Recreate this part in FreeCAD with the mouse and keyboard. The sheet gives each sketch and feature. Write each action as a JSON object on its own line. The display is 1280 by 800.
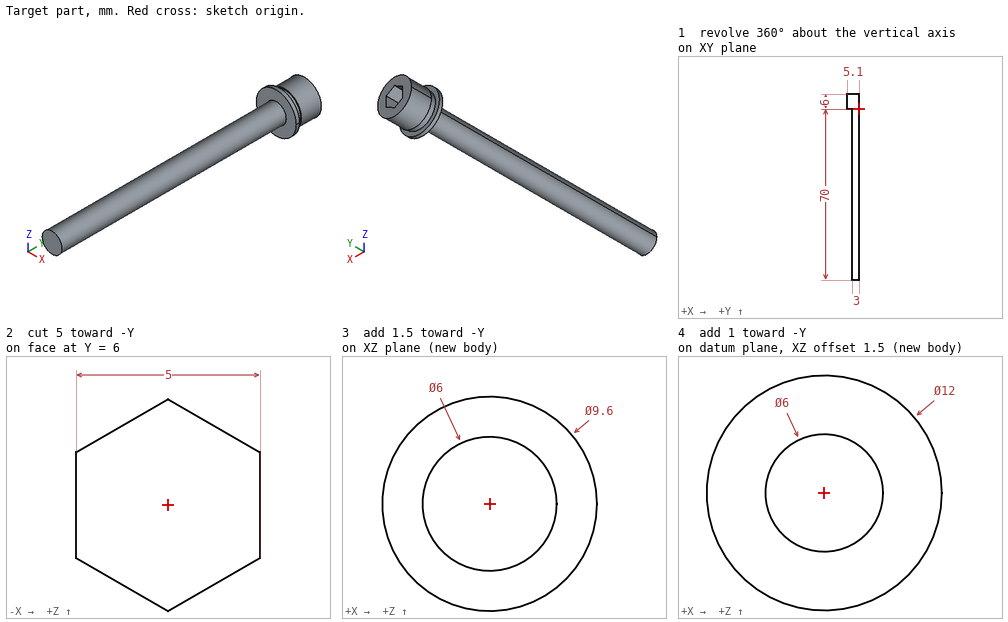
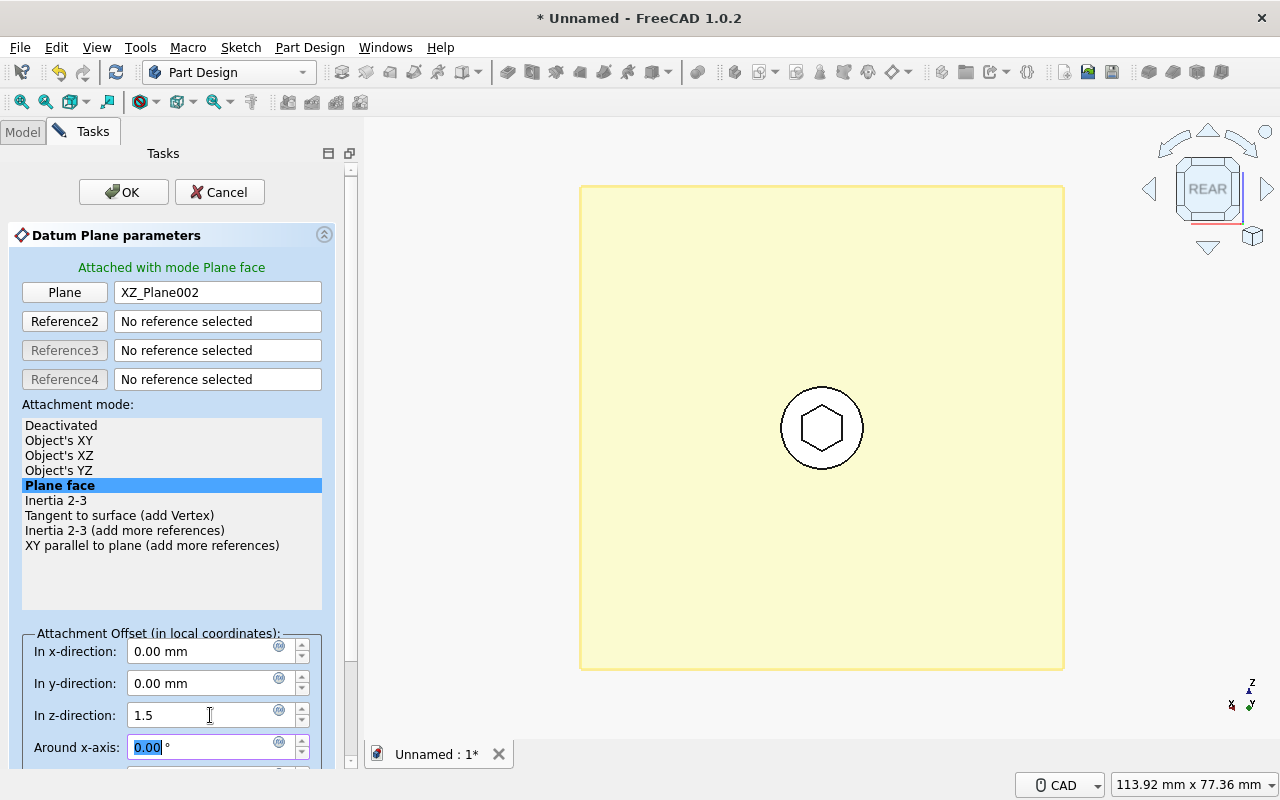
{"action": "left_click", "coordinate": [124, 192]}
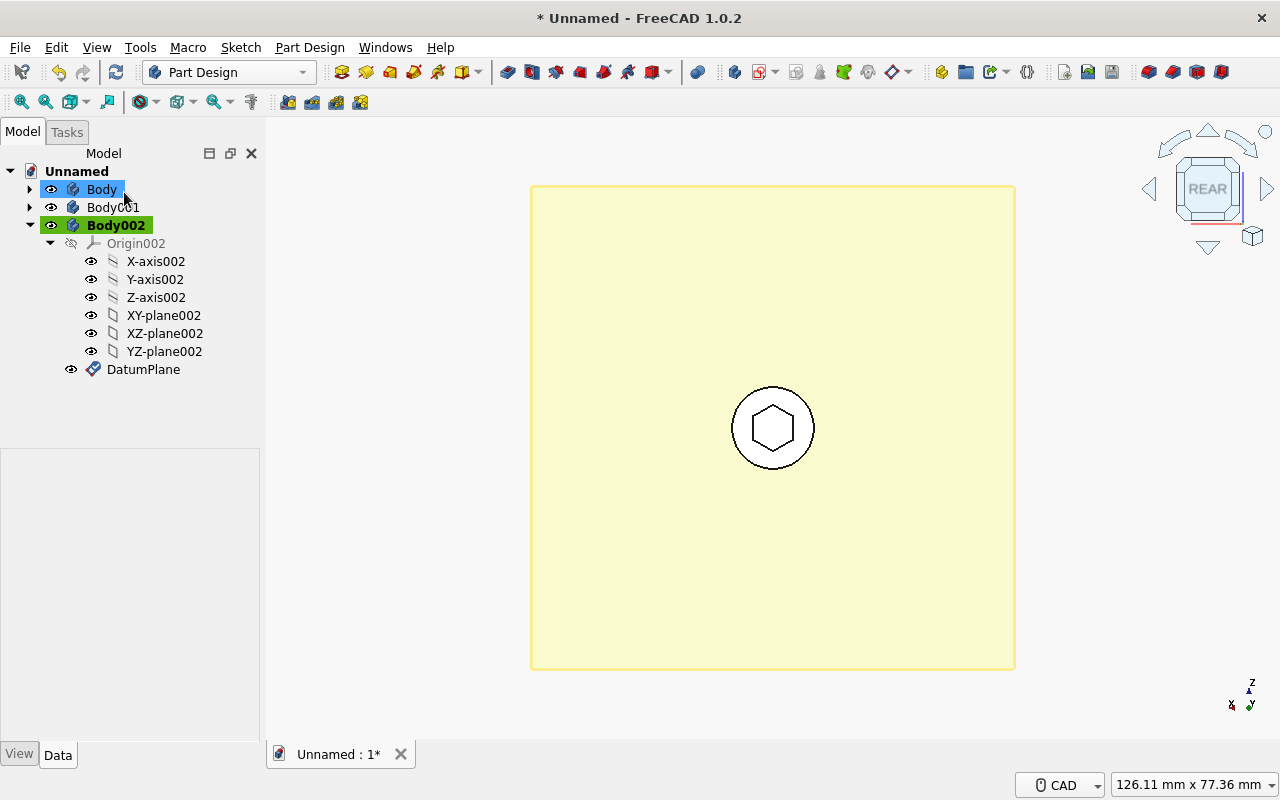
{"action": "left_click", "coordinate": [116, 369]}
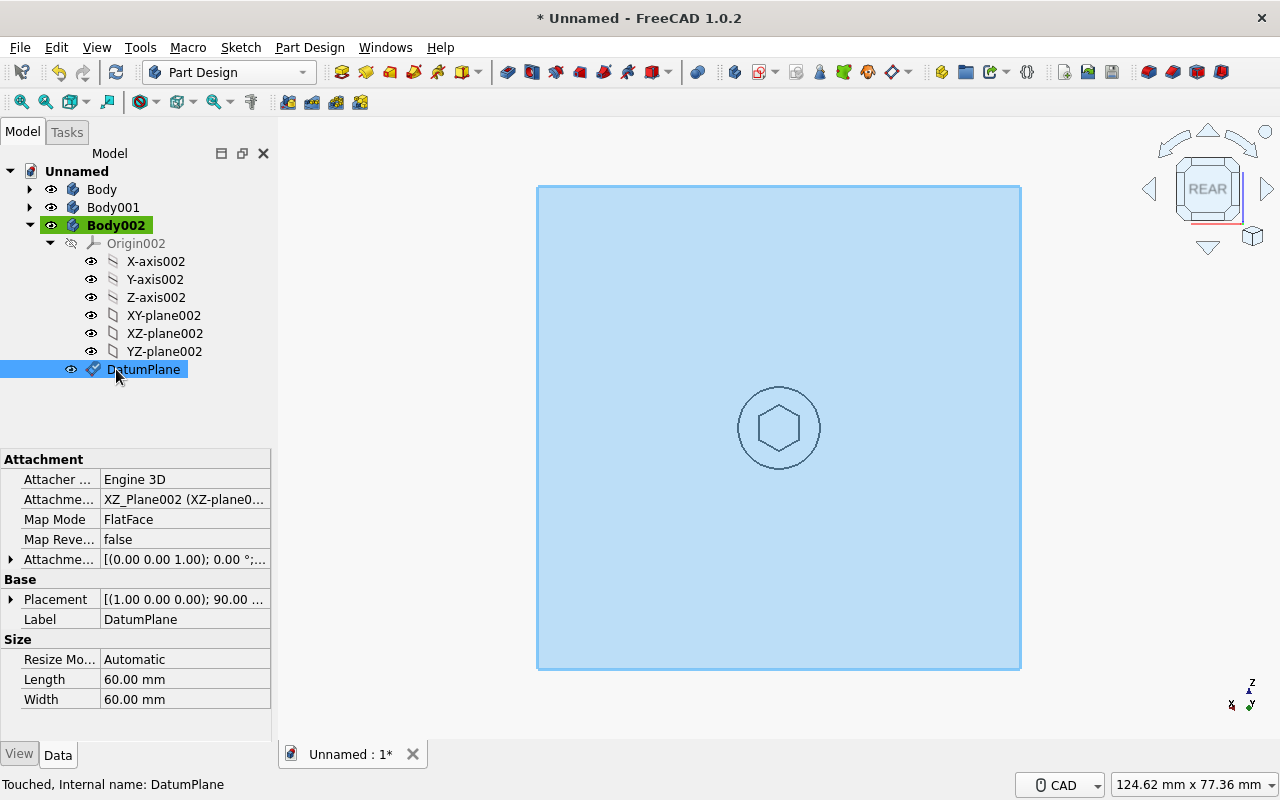
{"action": "left_click", "coordinate": [760, 72]}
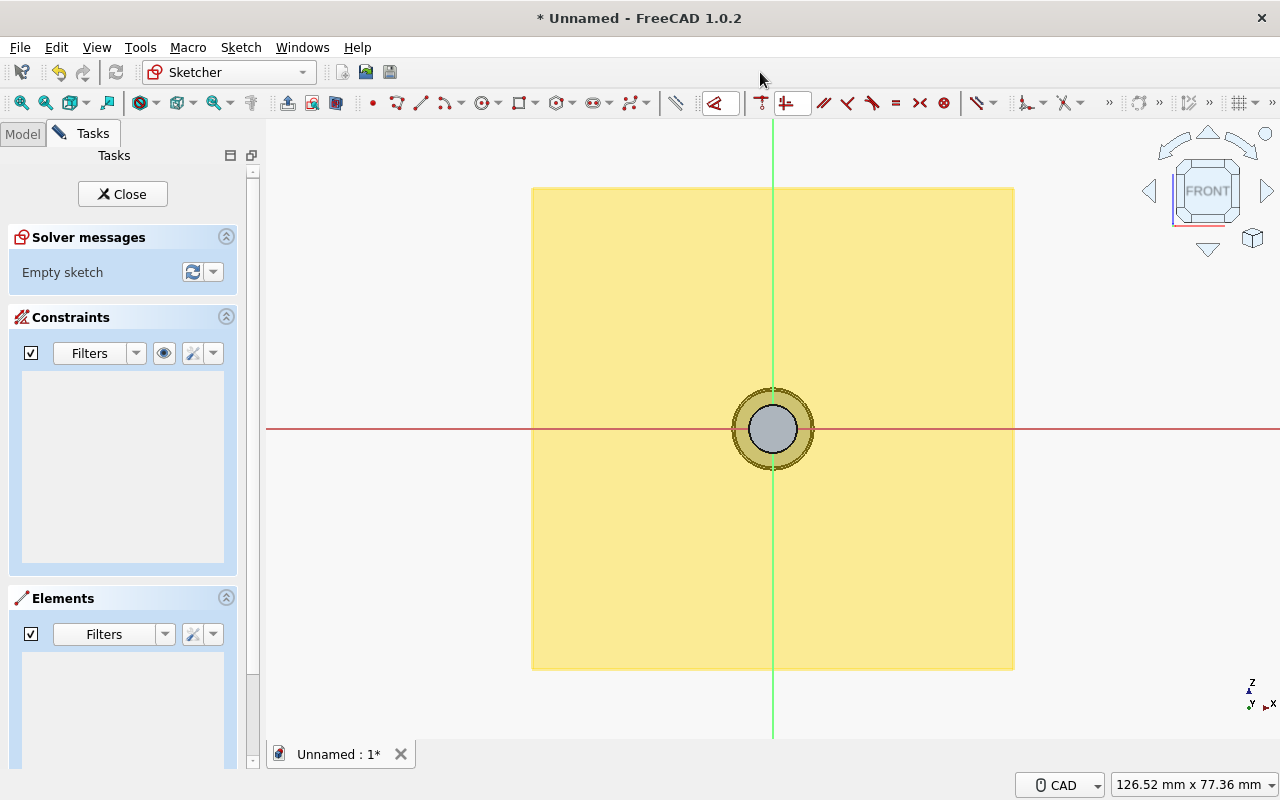
{"action": "scroll", "coordinate": [795, 429], "scroll_direction": "up", "scroll_amount": 7}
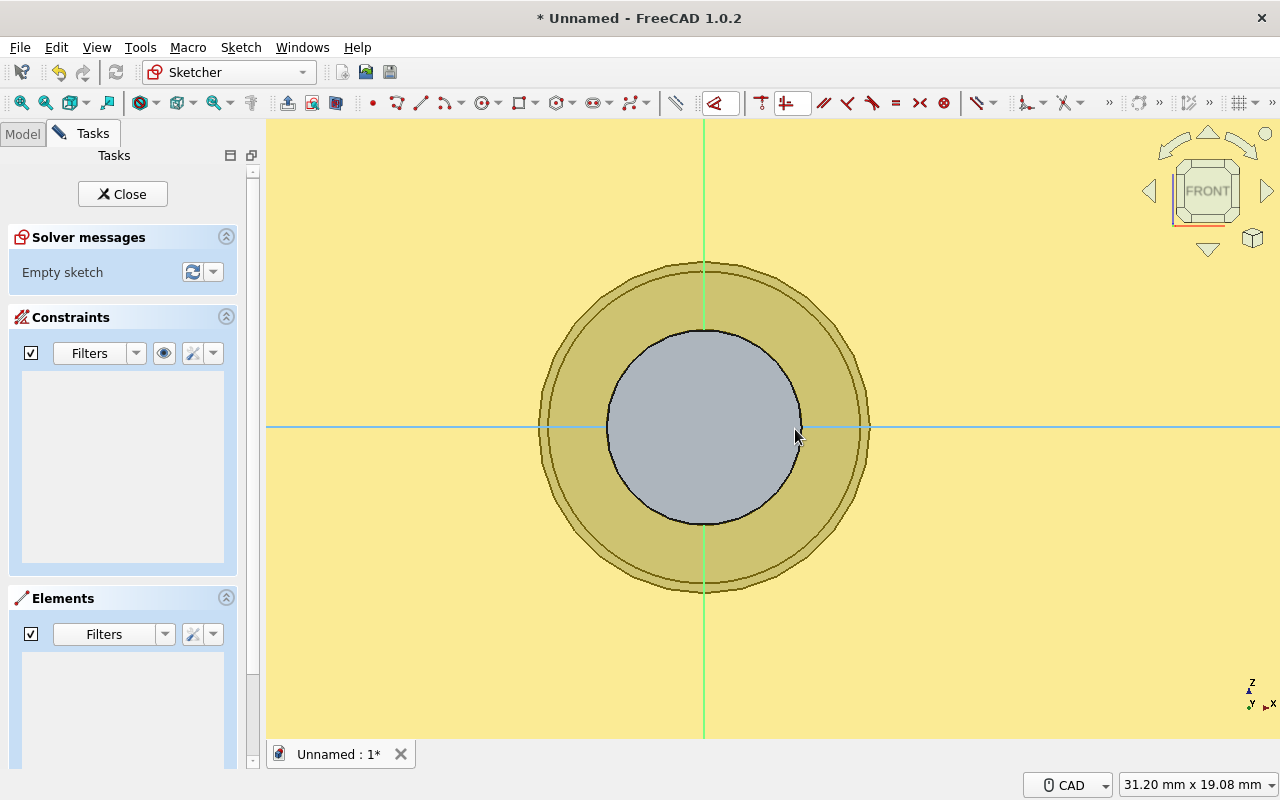
{"action": "key", "text": "g c"}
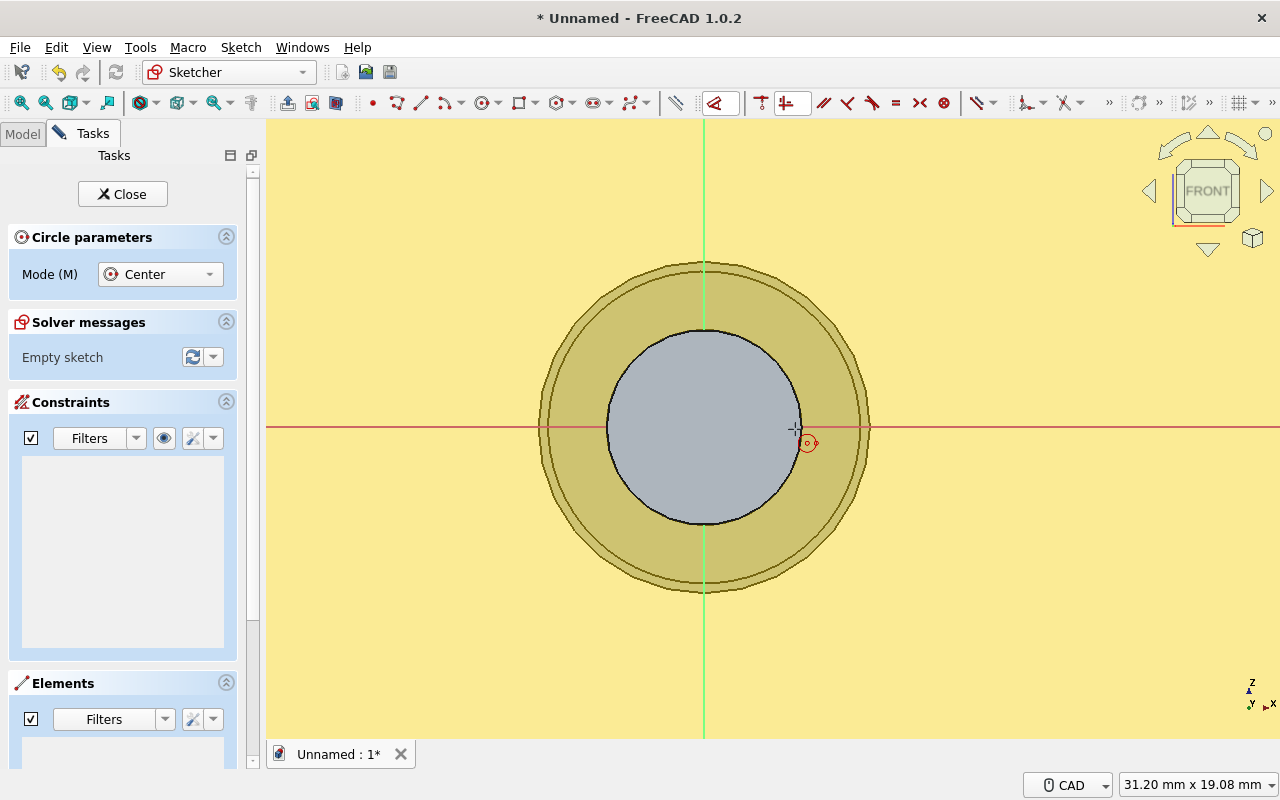
{"action": "left_click", "coordinate": [704, 427]}
{"action": "left_click", "coordinate": [842, 290]}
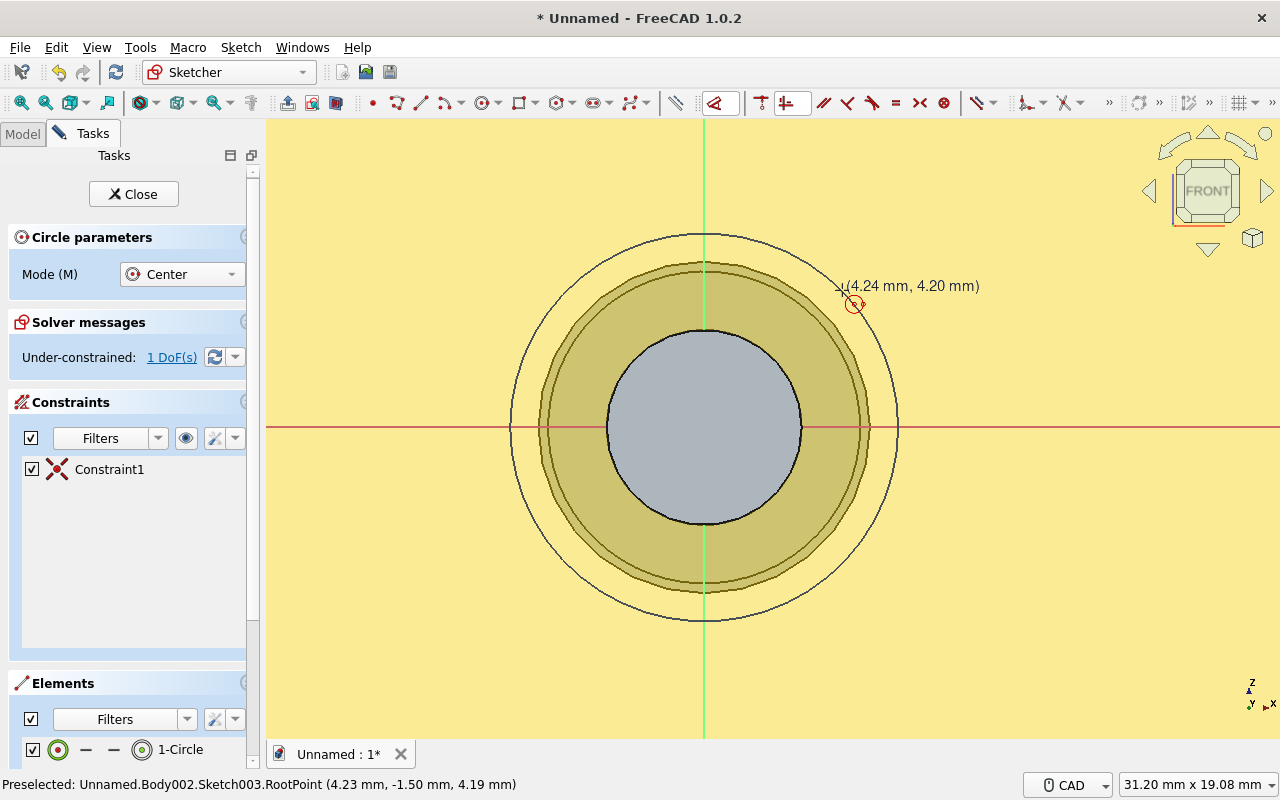
{"action": "left_click", "coordinate": [704, 427]}
{"action": "left_click", "coordinate": [773, 359]}
{"action": "key", "text": "Escape"}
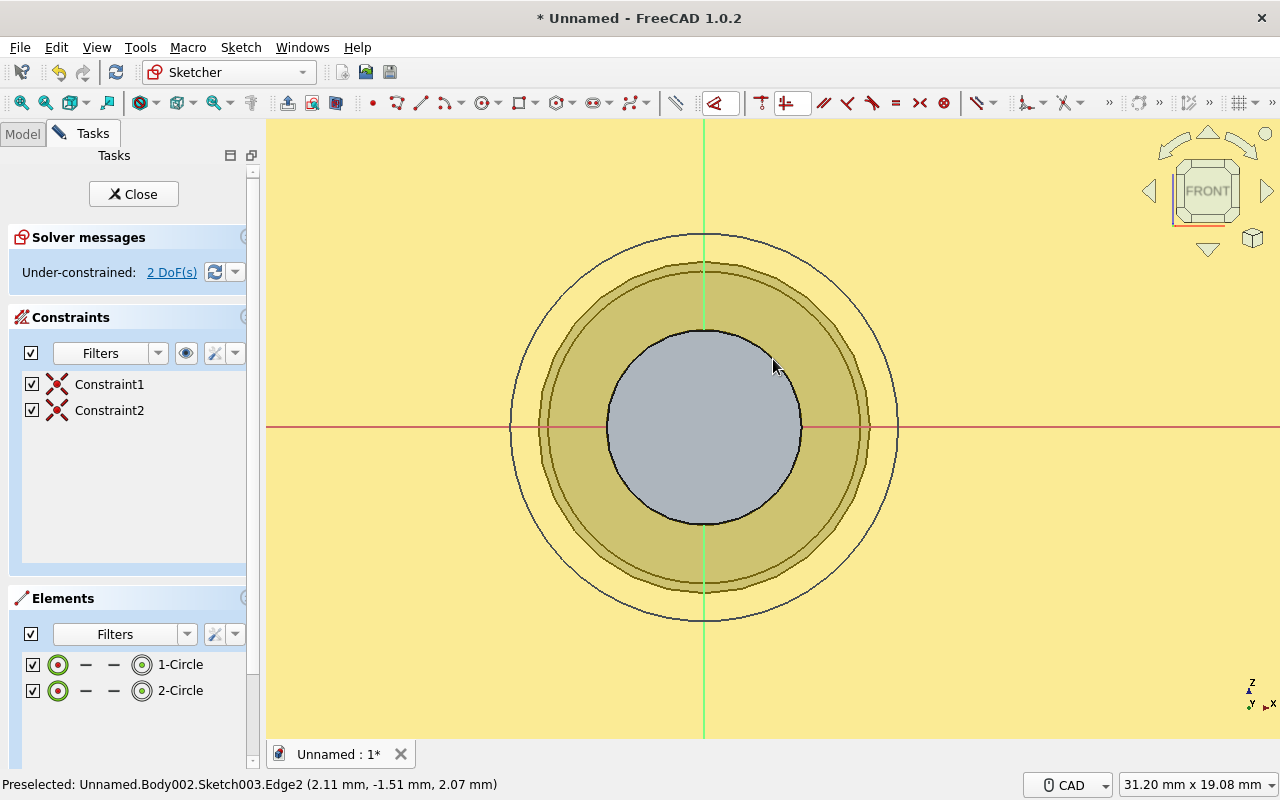
{"action": "left_click", "coordinate": [841, 290]}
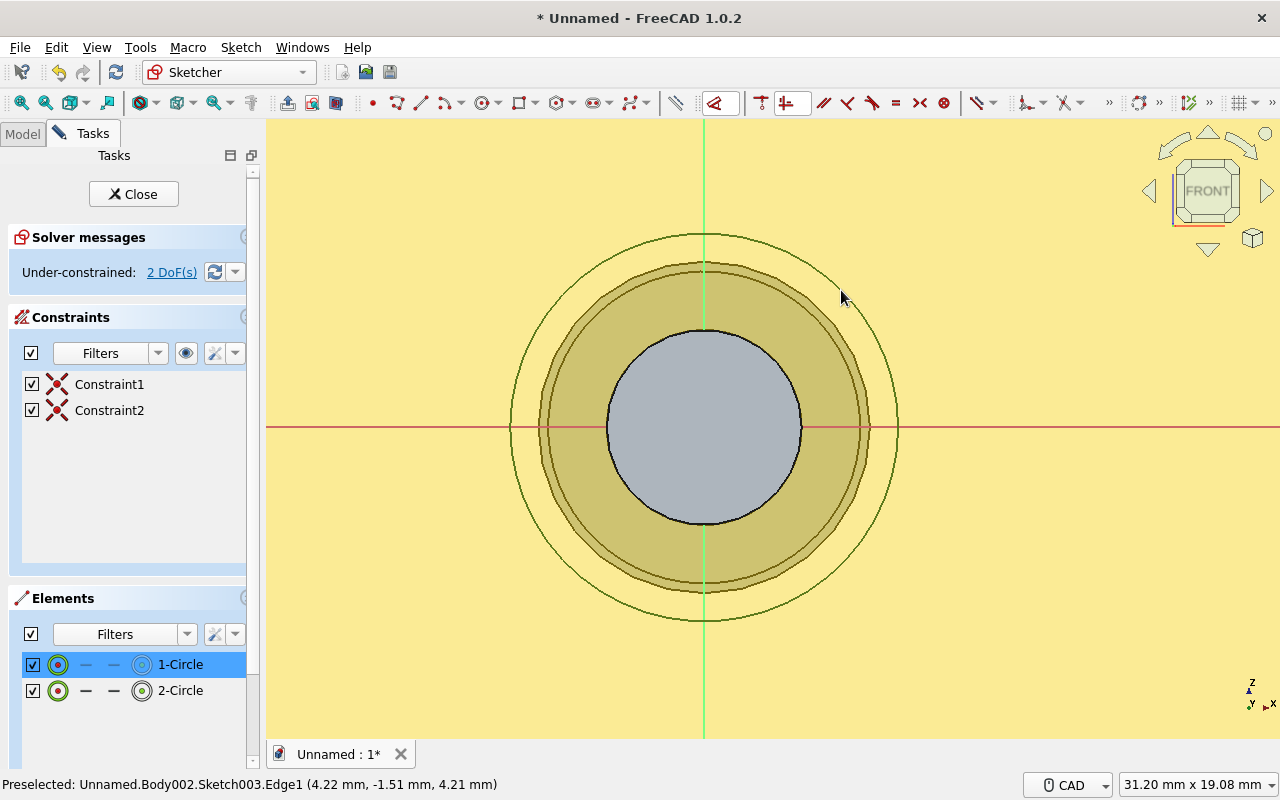
{"action": "key", "text": "k o"}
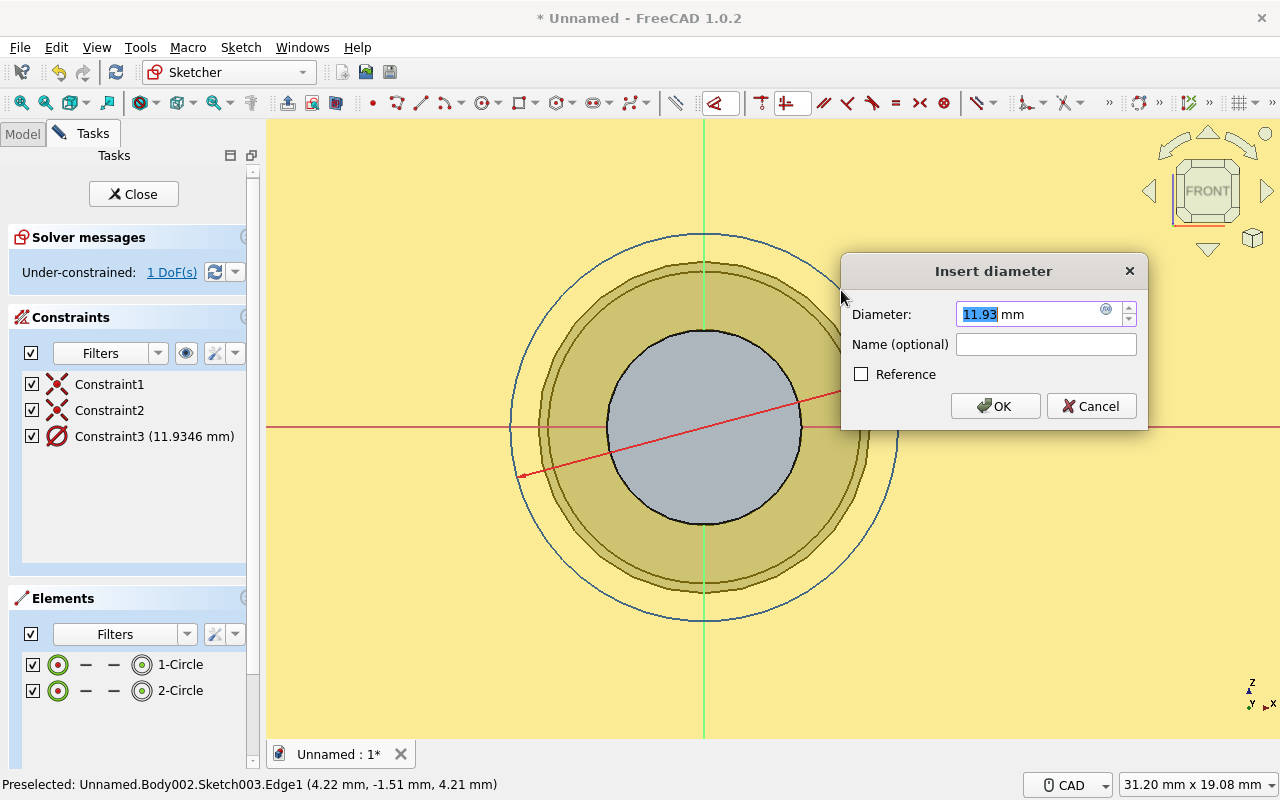
{"action": "type", "text": "12"}
{"action": "key", "text": "Return"}